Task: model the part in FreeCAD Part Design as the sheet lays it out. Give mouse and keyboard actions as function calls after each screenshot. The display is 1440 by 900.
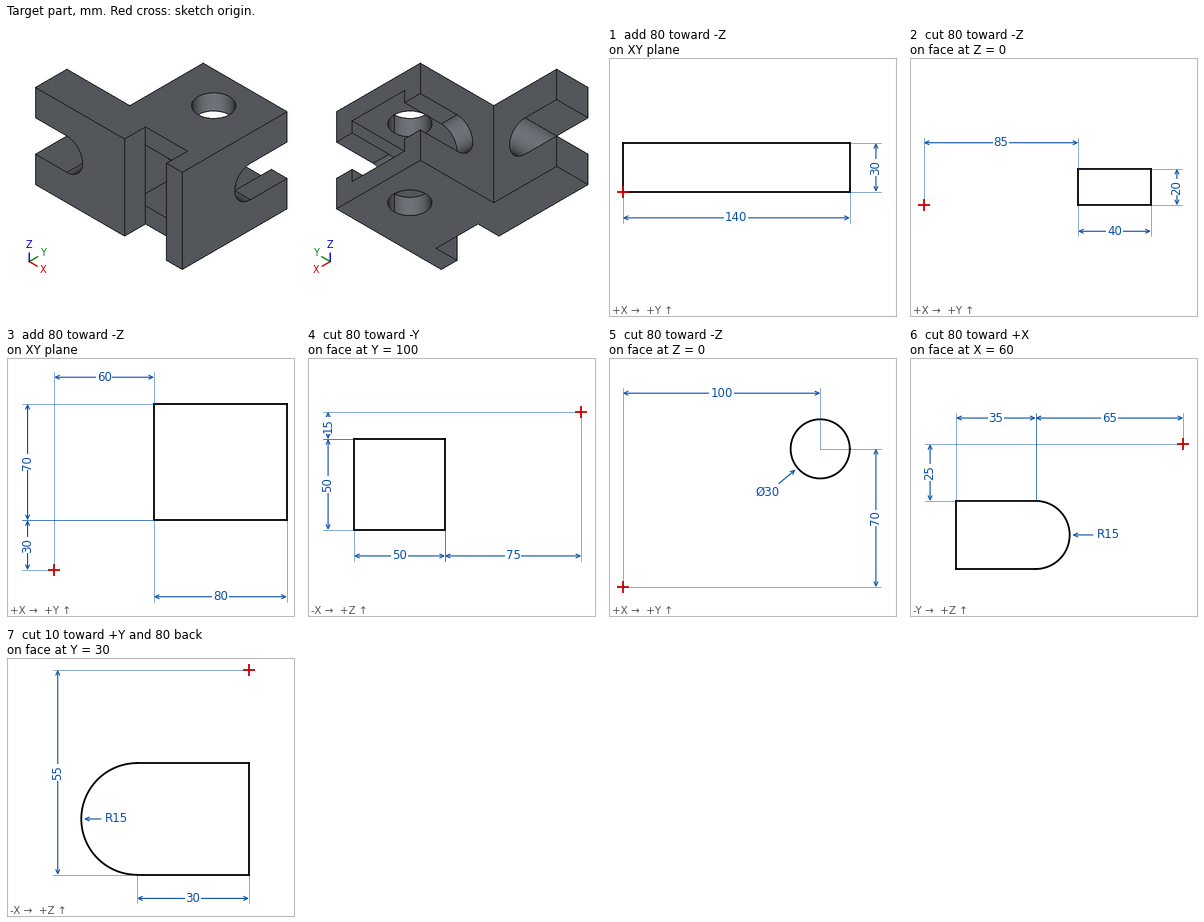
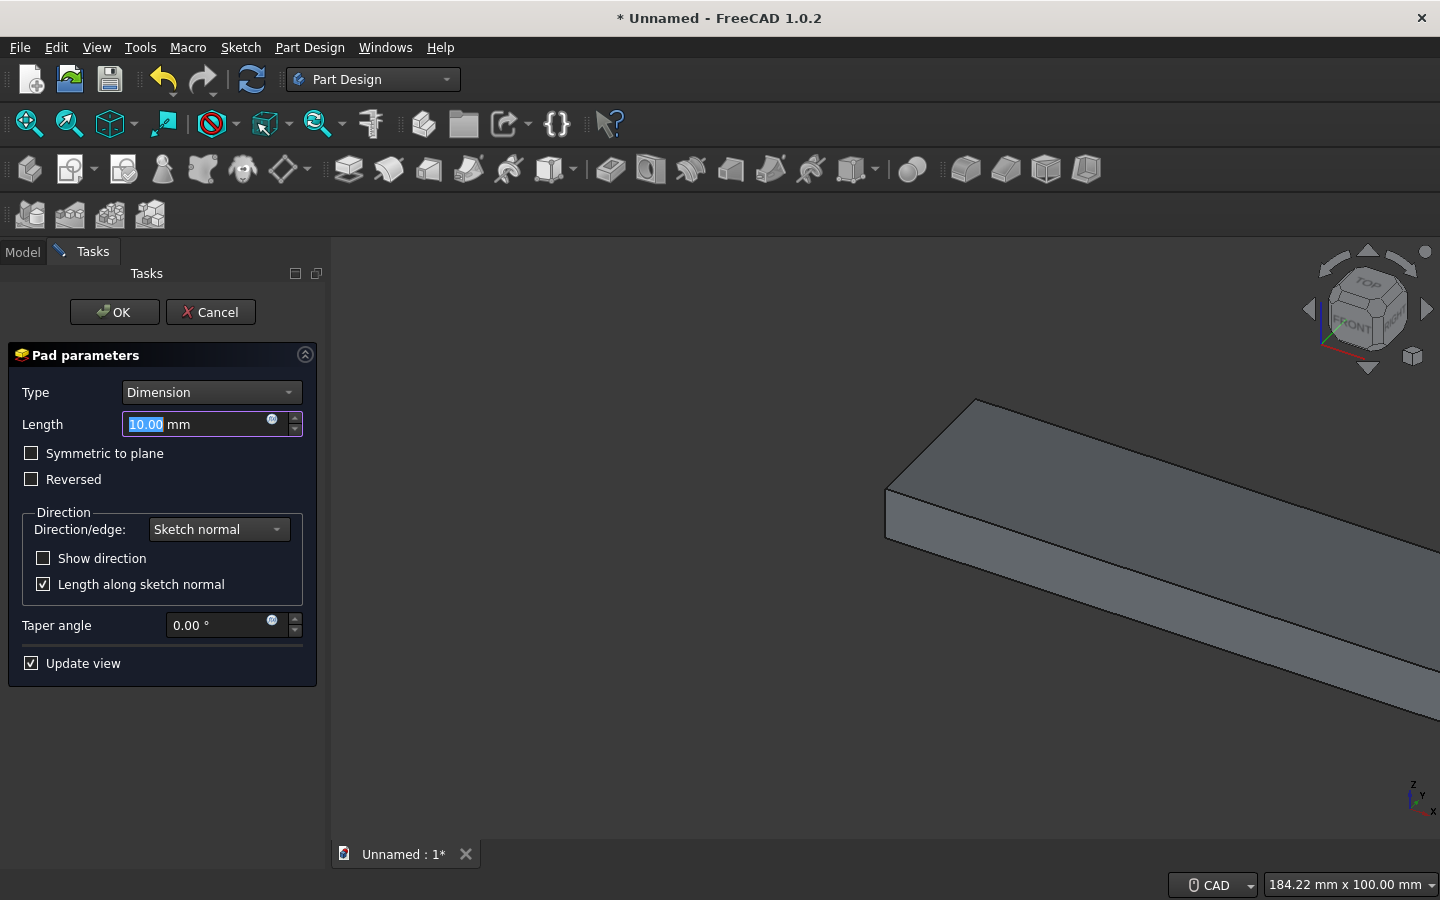
text(80)
key(Tab)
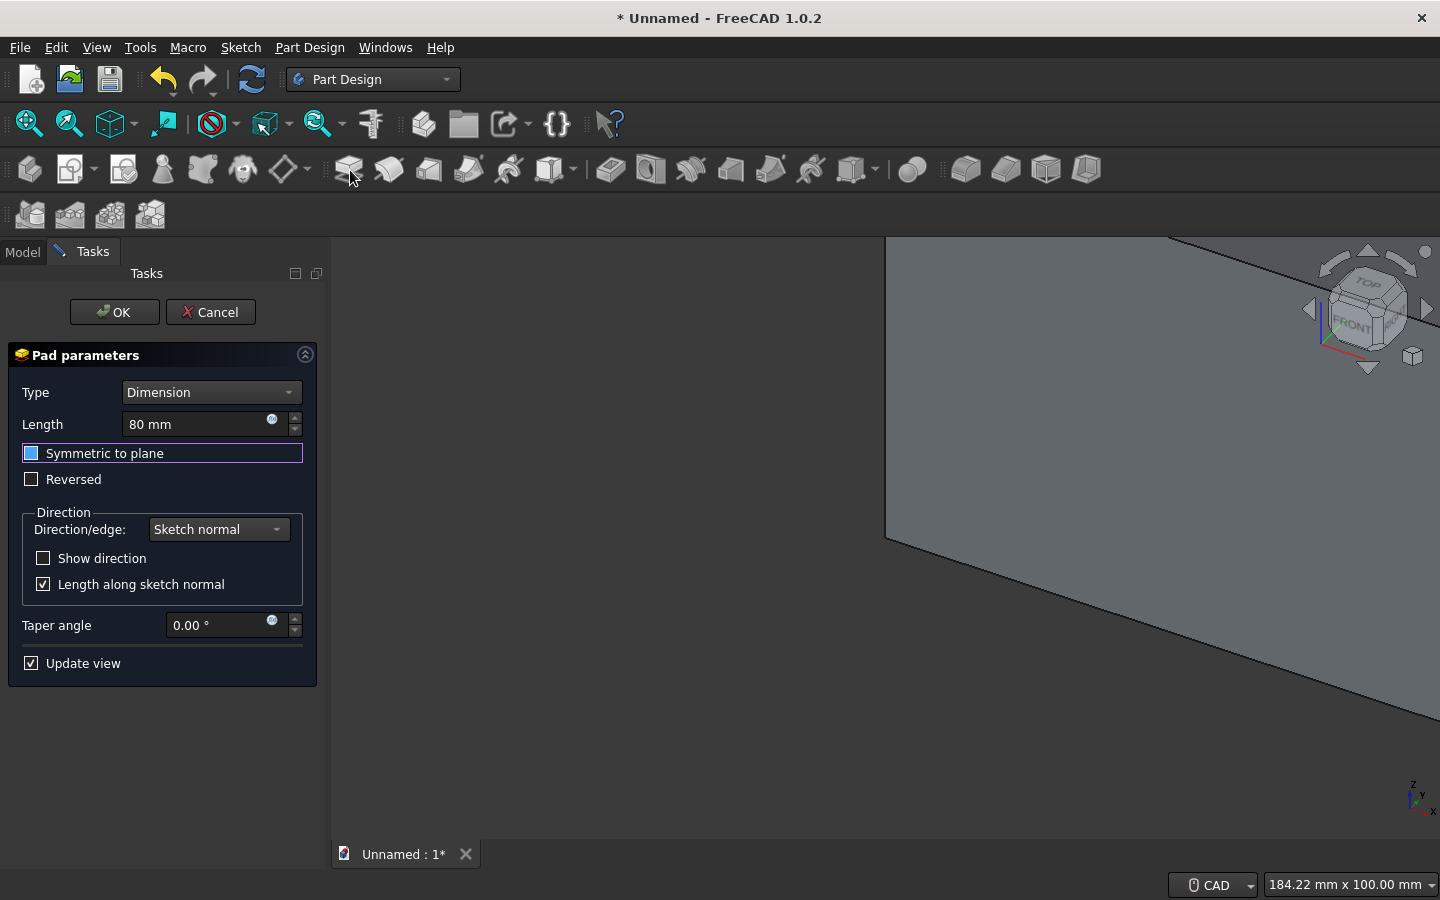
click(30, 479)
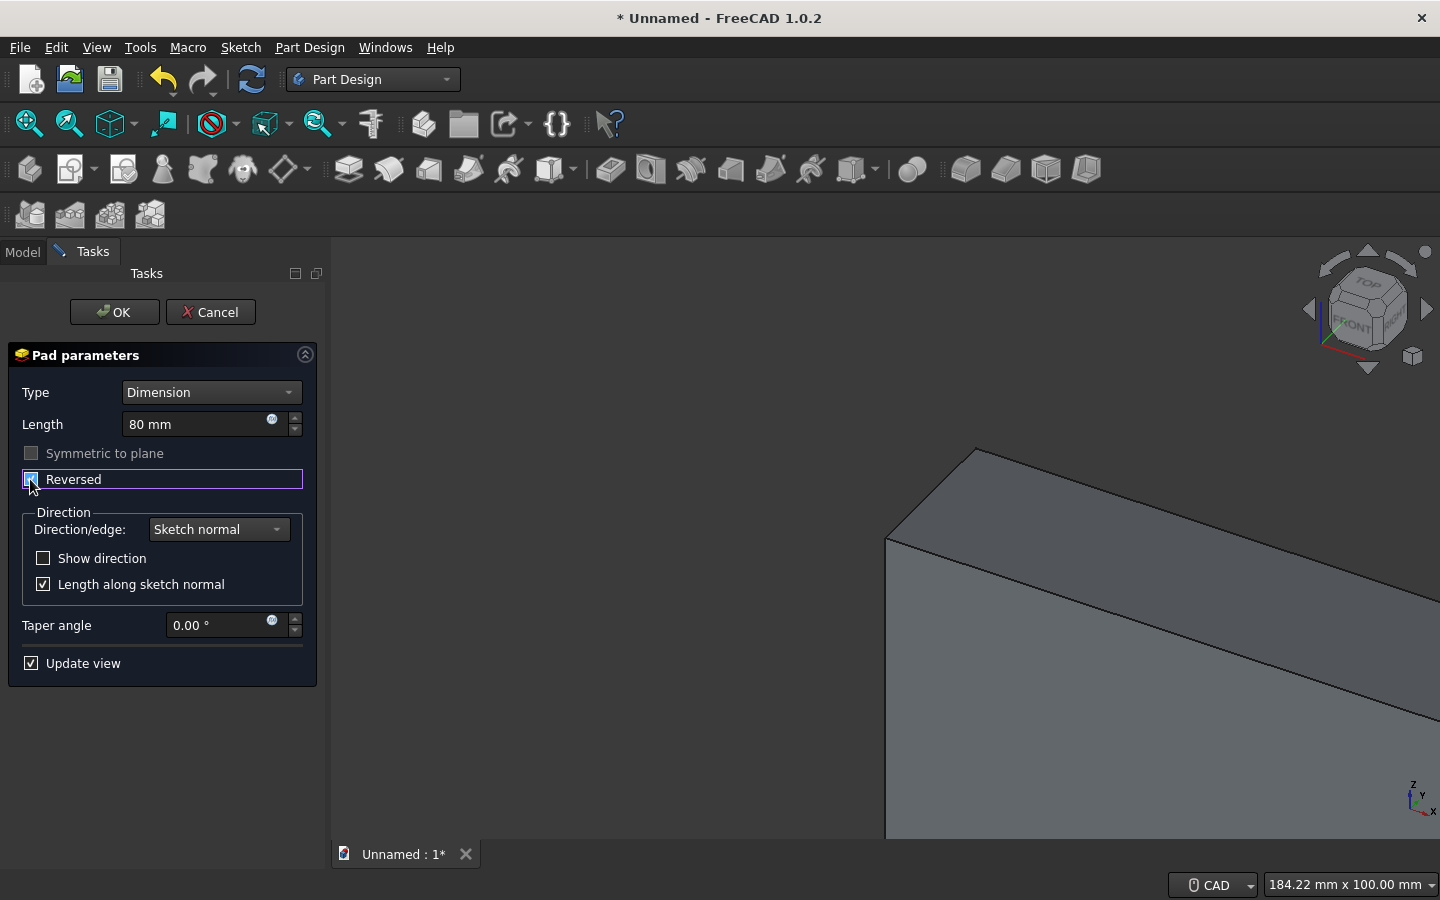
click(115, 312)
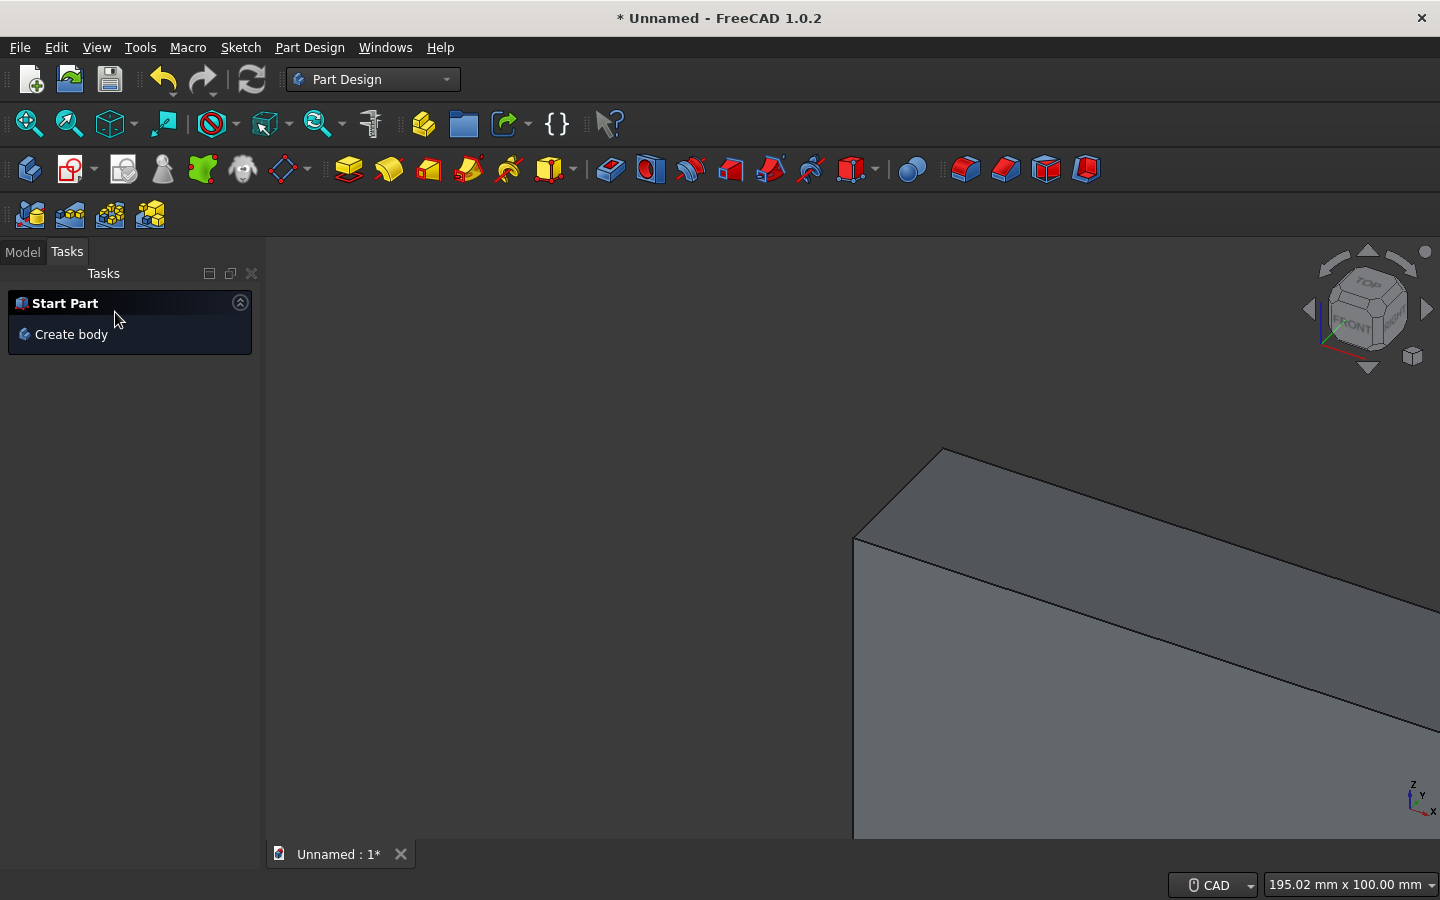
click(30, 124)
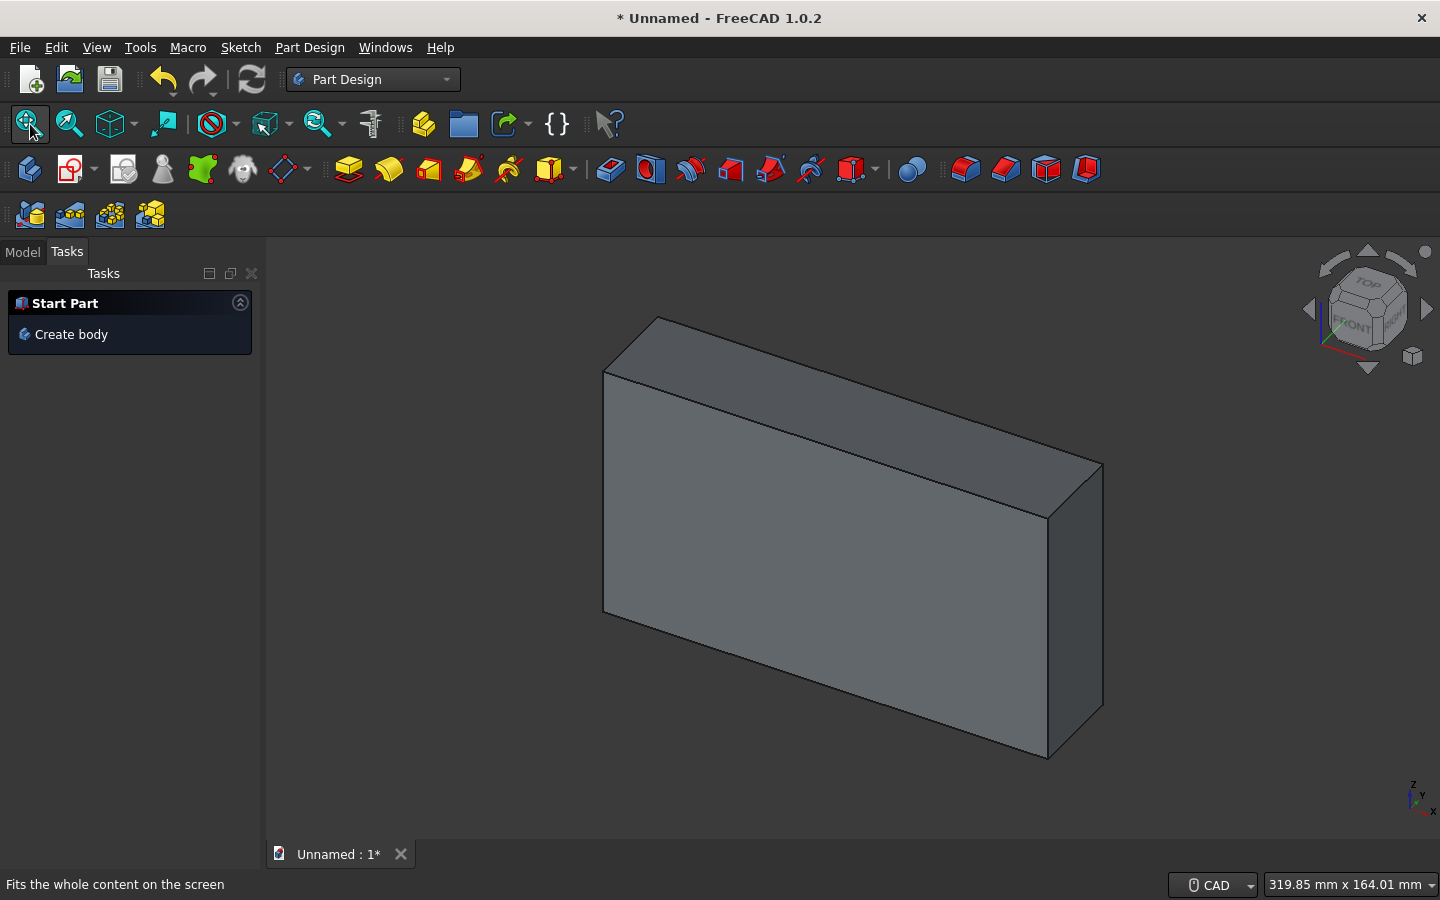
click(980, 459)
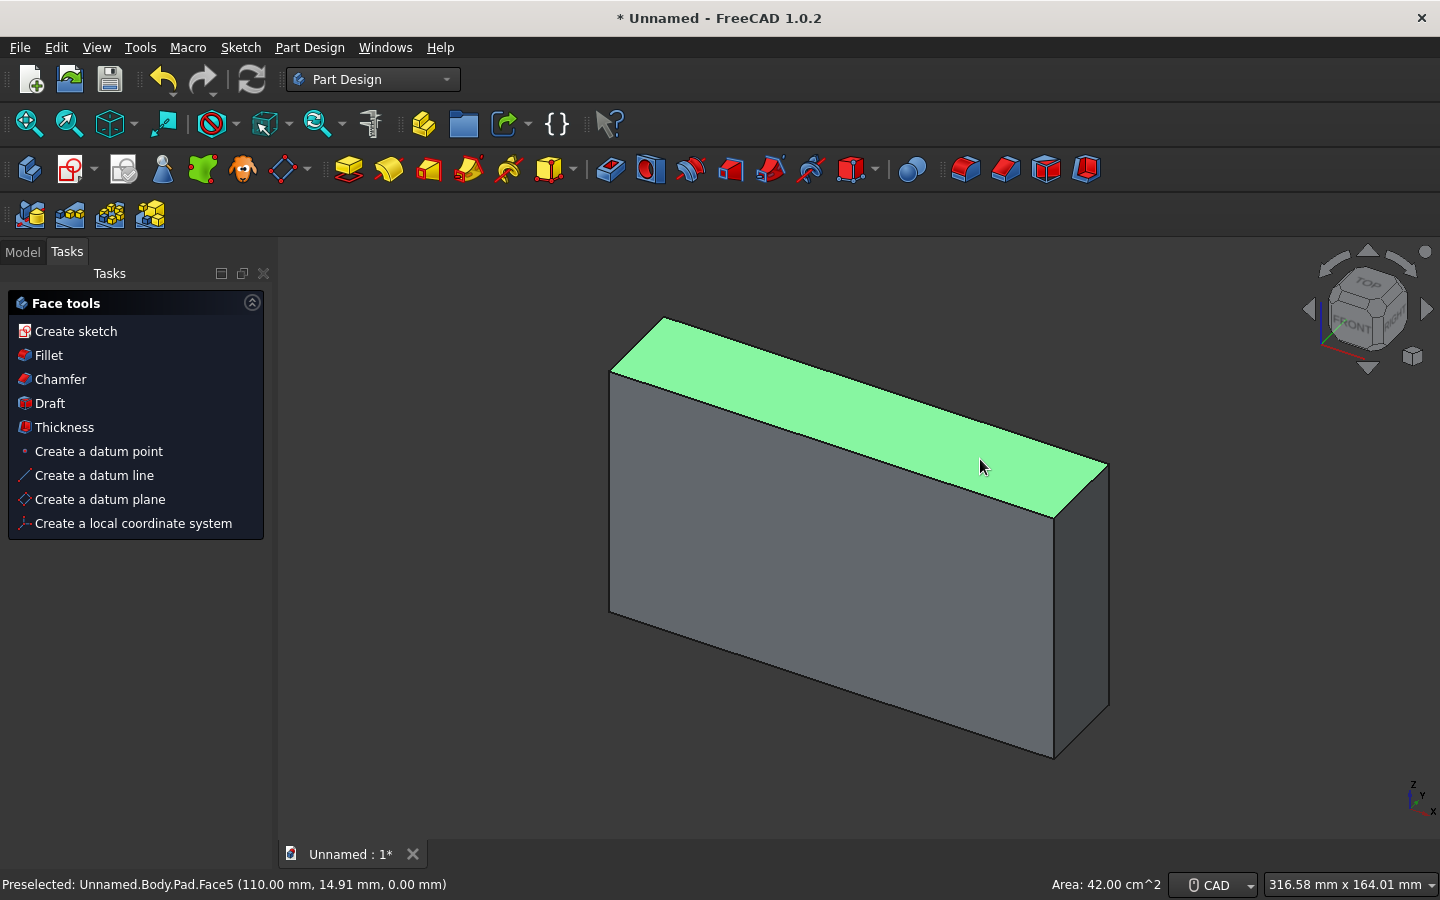
click(70, 170)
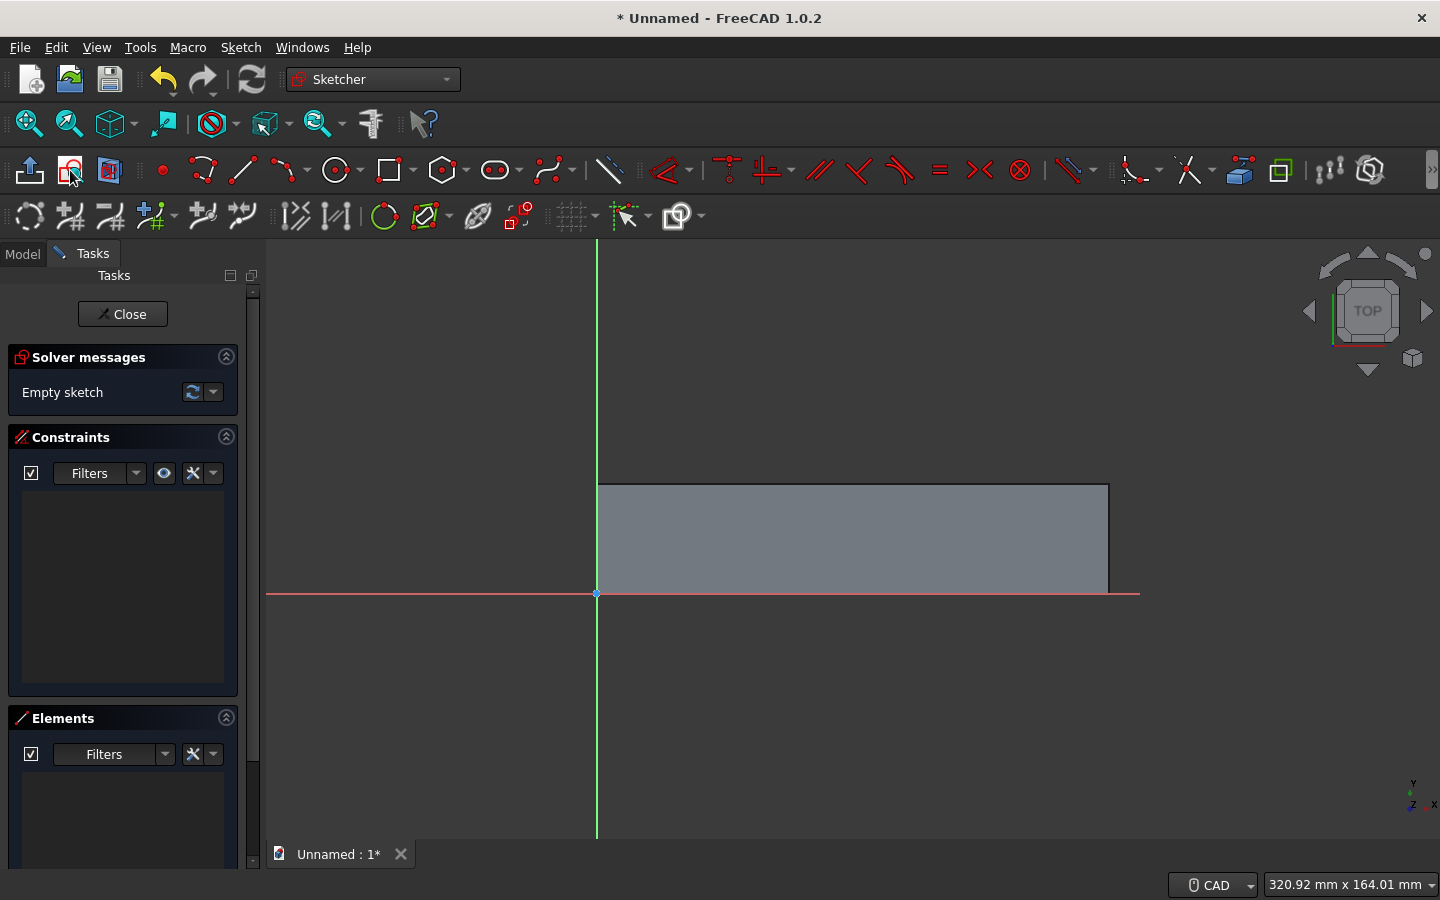
scroll(1031, 562, up, 8)